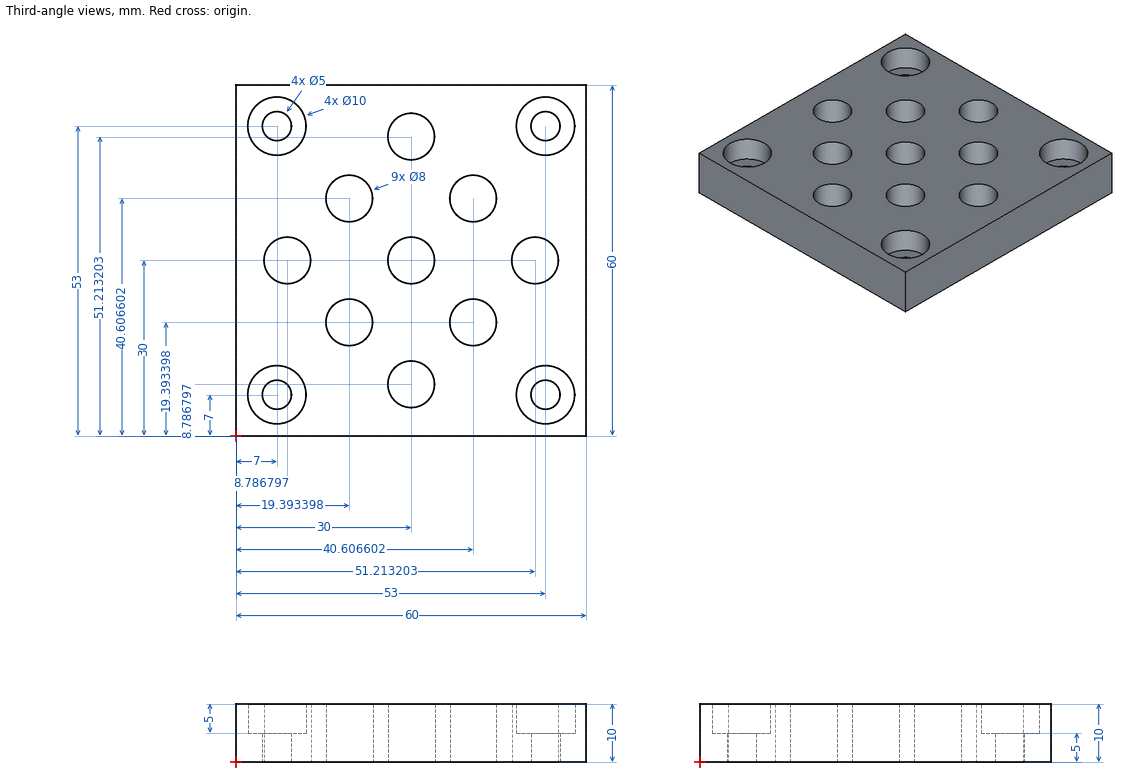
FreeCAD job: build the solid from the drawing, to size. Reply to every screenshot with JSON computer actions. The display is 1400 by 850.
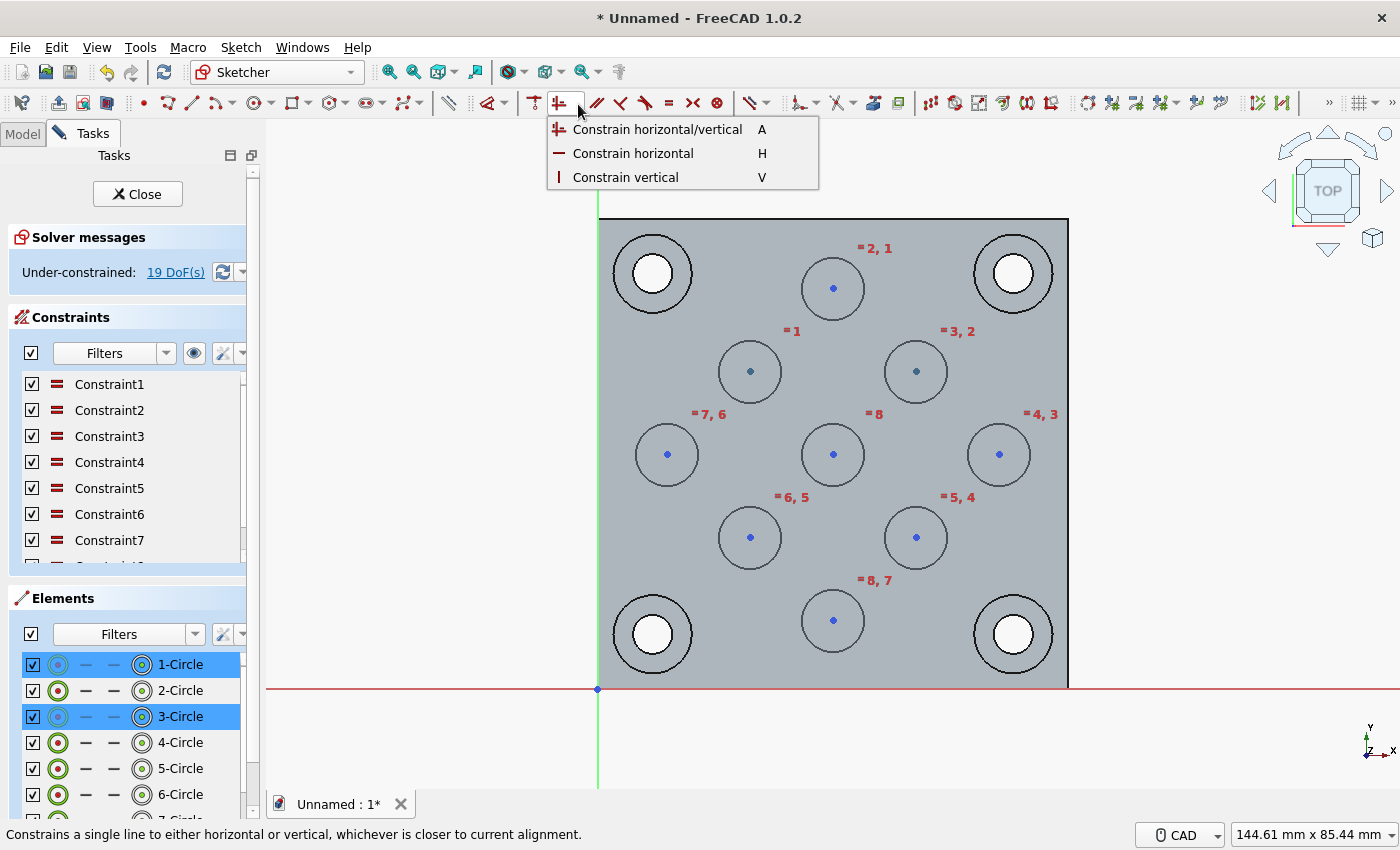
{"action": "left_click", "coordinate": [683, 153]}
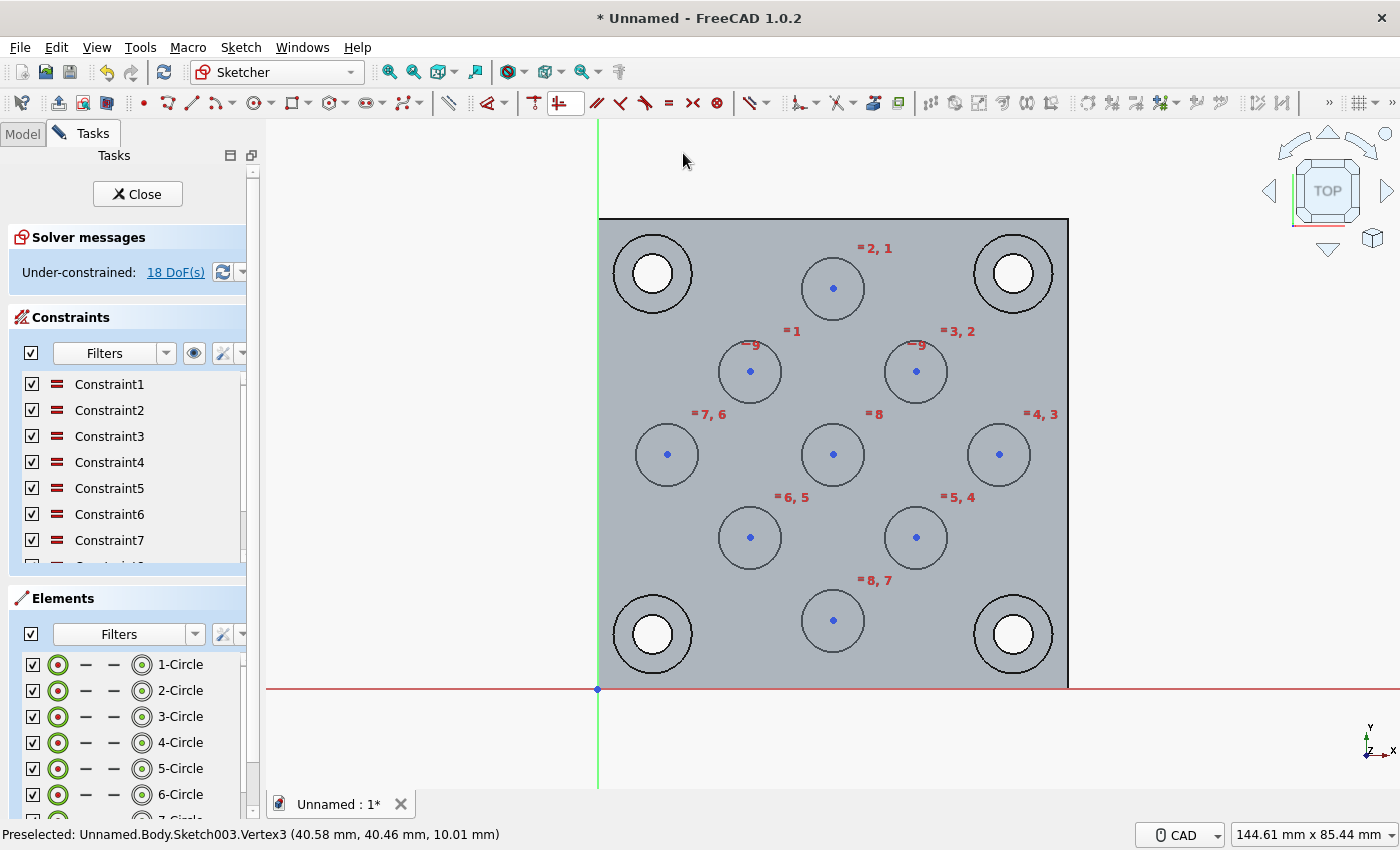
{"action": "left_click", "coordinate": [916, 372]}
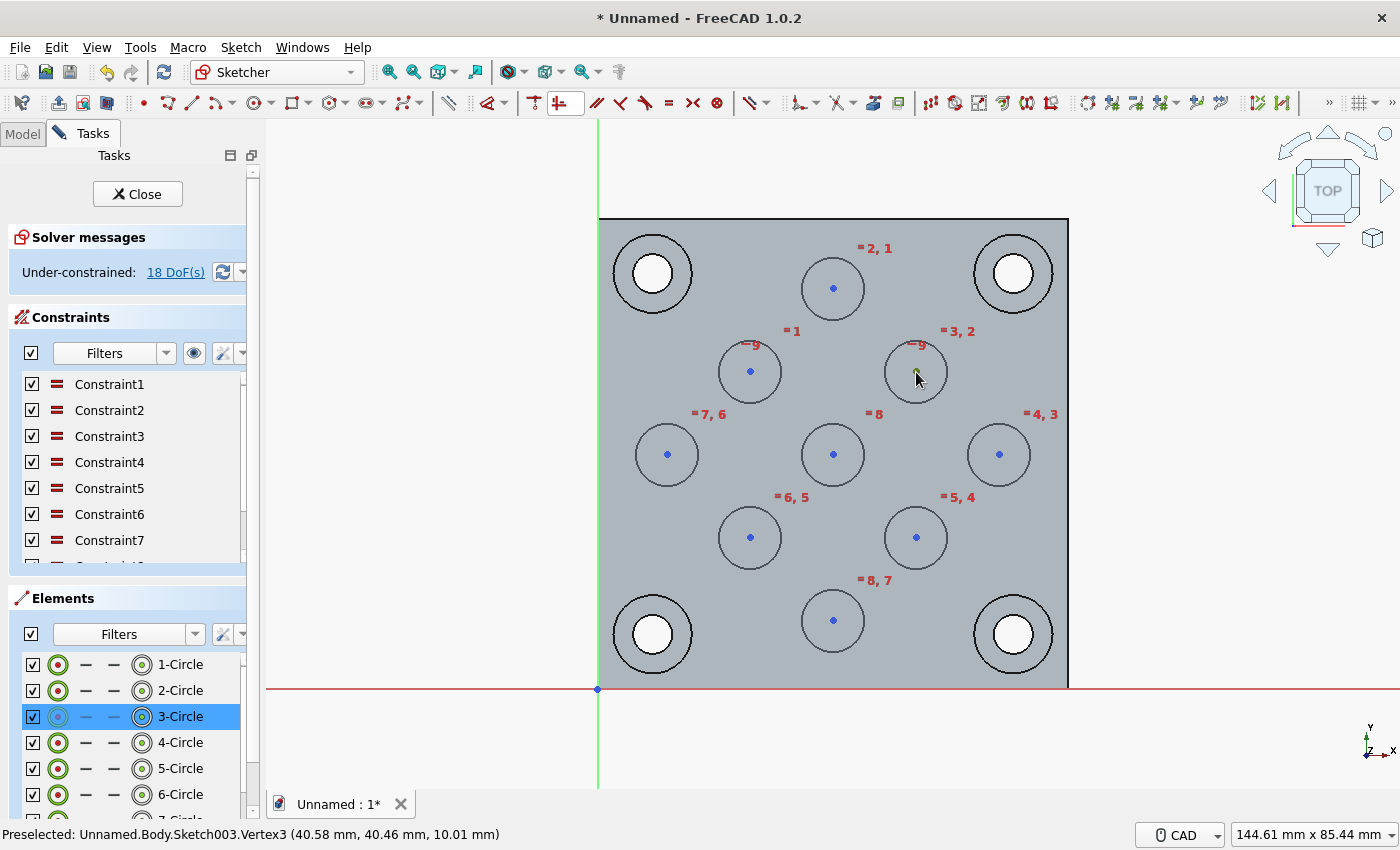
{"action": "left_click", "coordinate": [916, 538]}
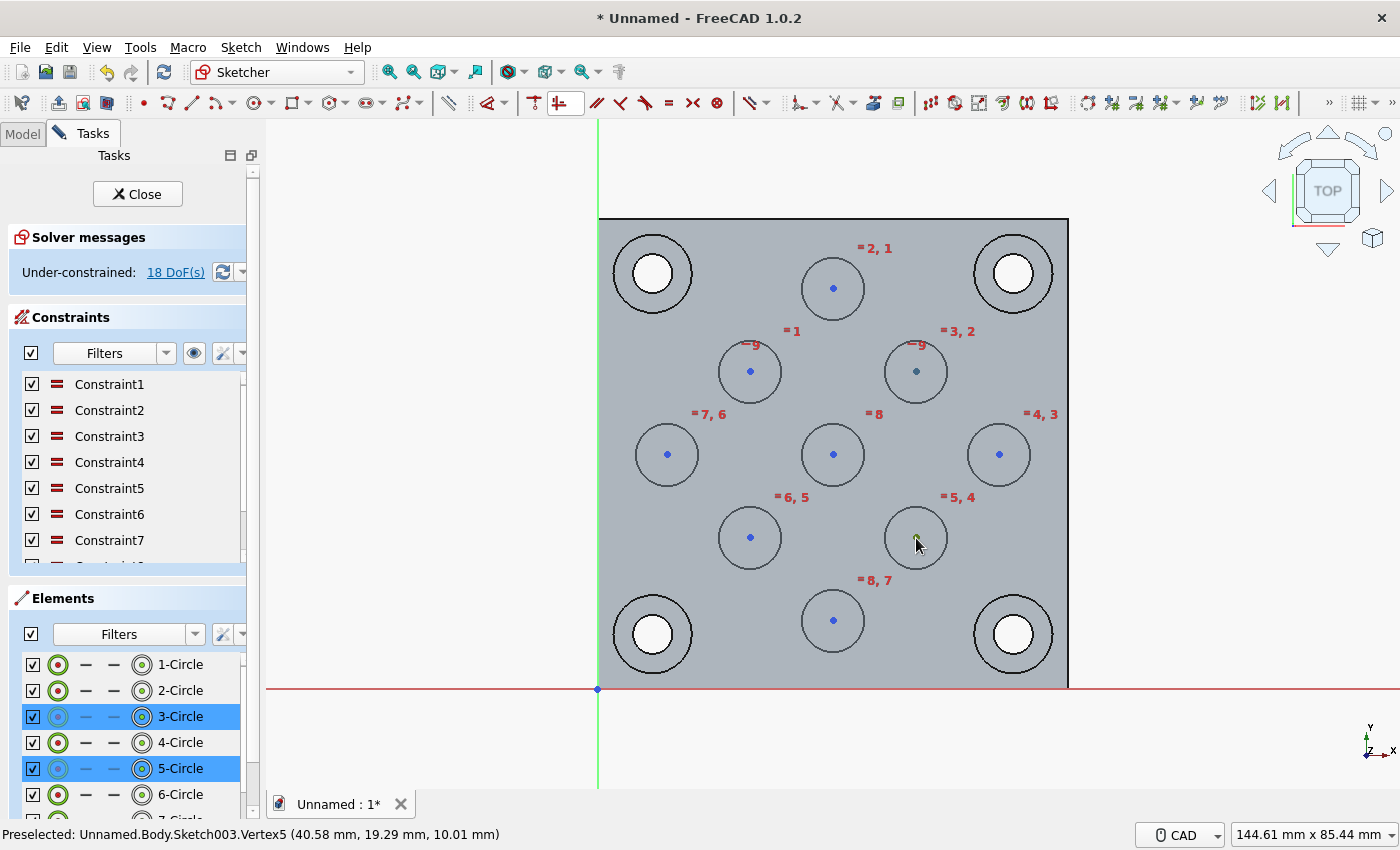
{"action": "left_click", "coordinate": [578, 104]}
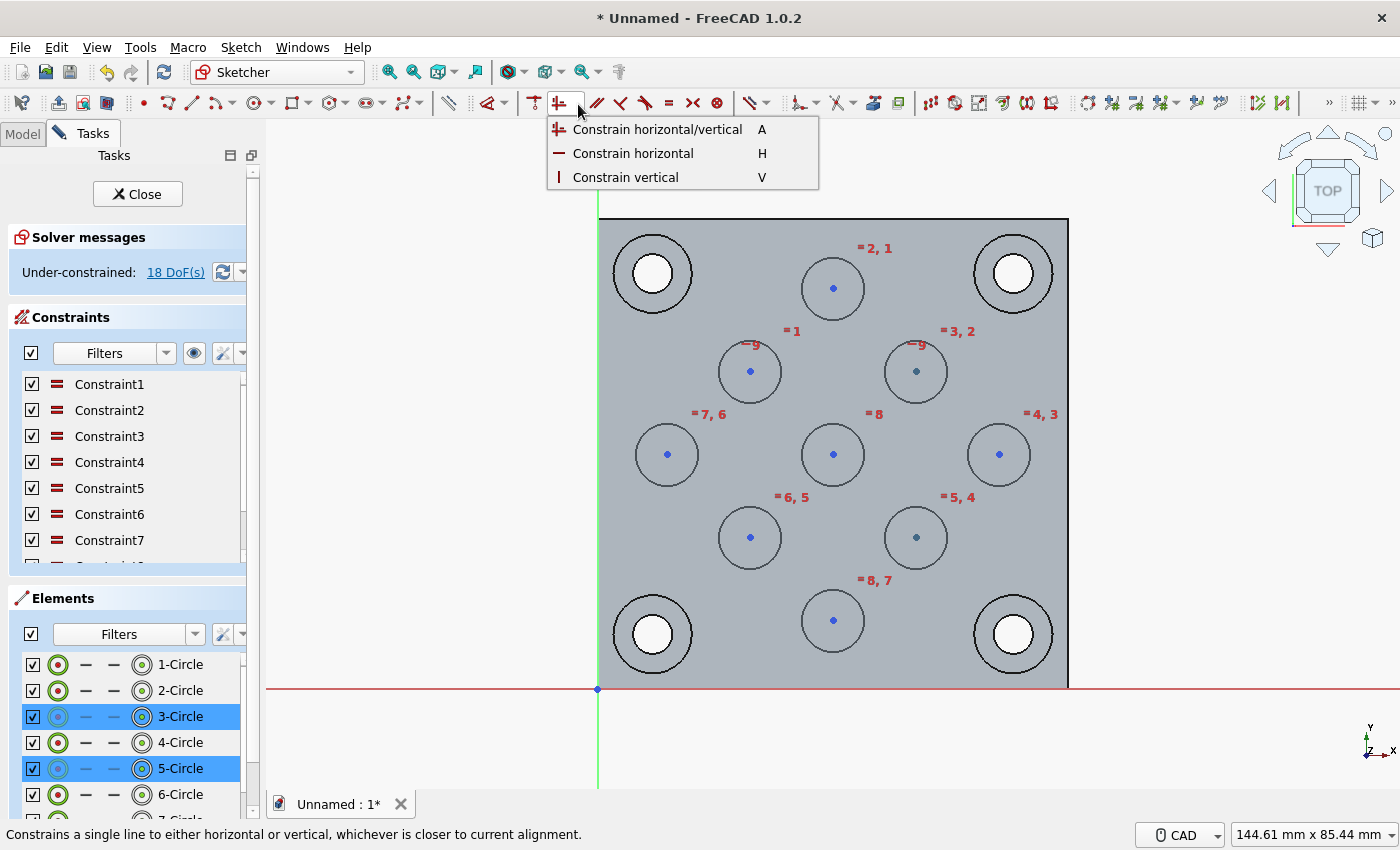
{"action": "left_click", "coordinate": [683, 177]}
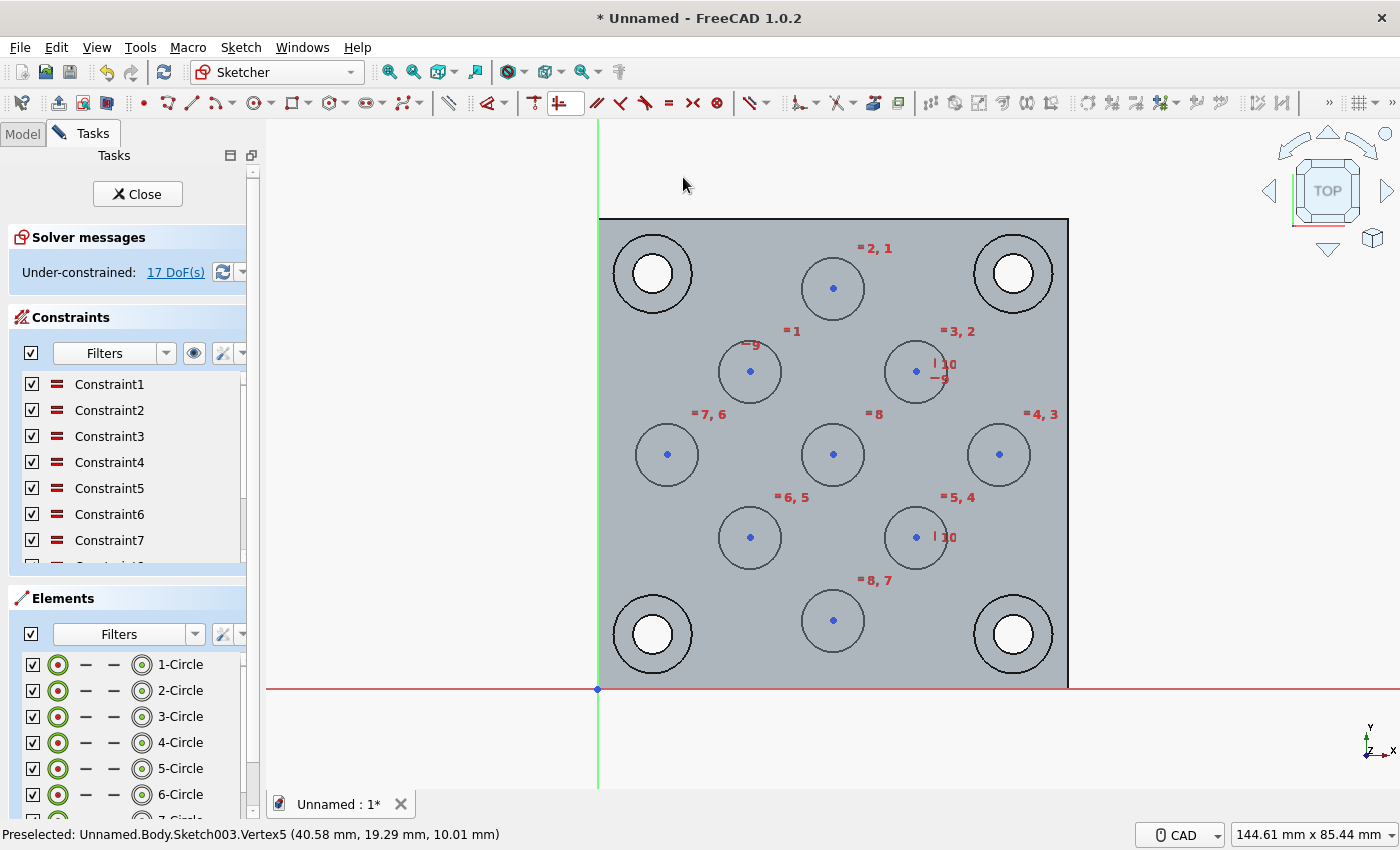
{"action": "left_click", "coordinate": [750, 372]}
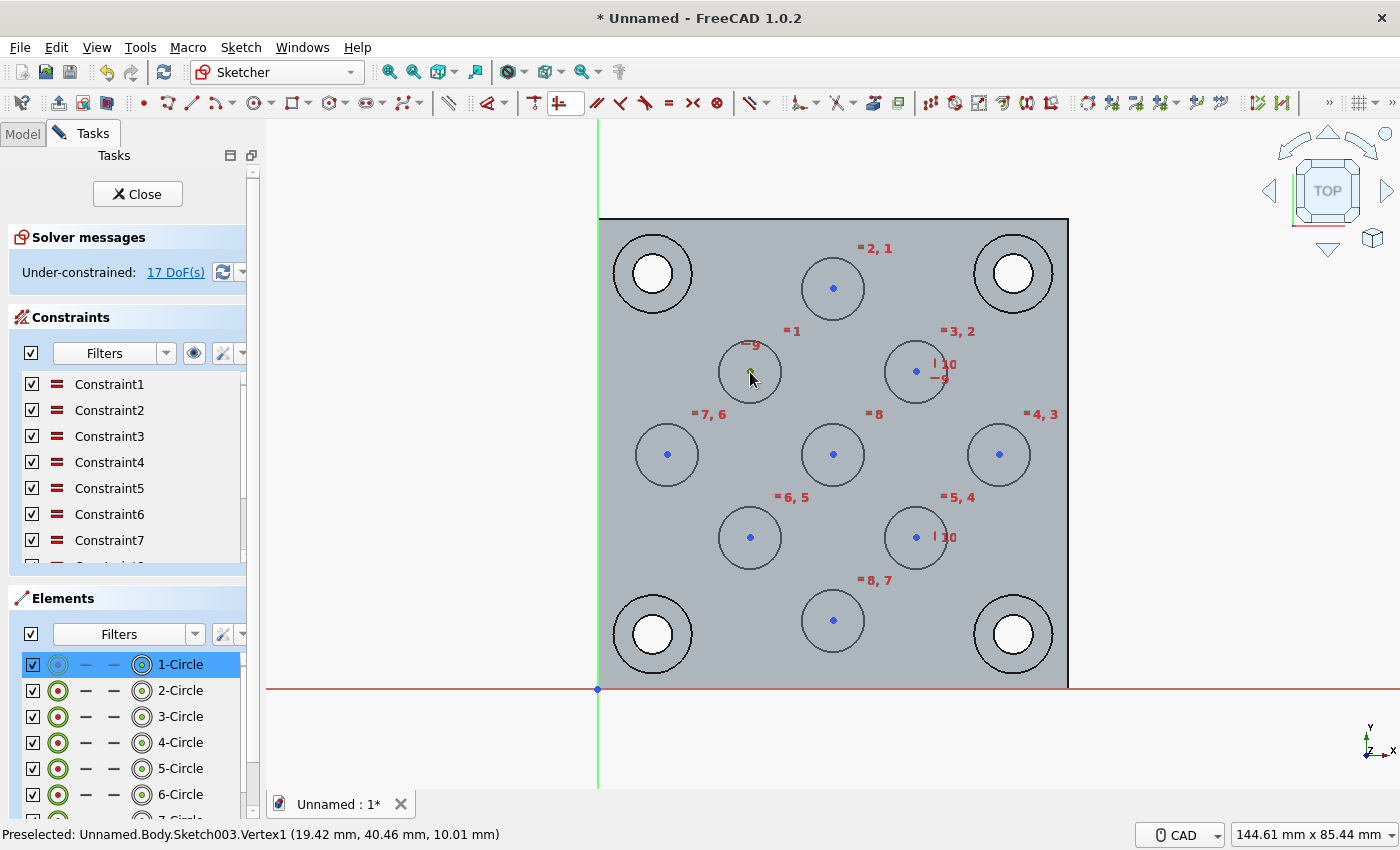
{"action": "left_click", "coordinate": [750, 538]}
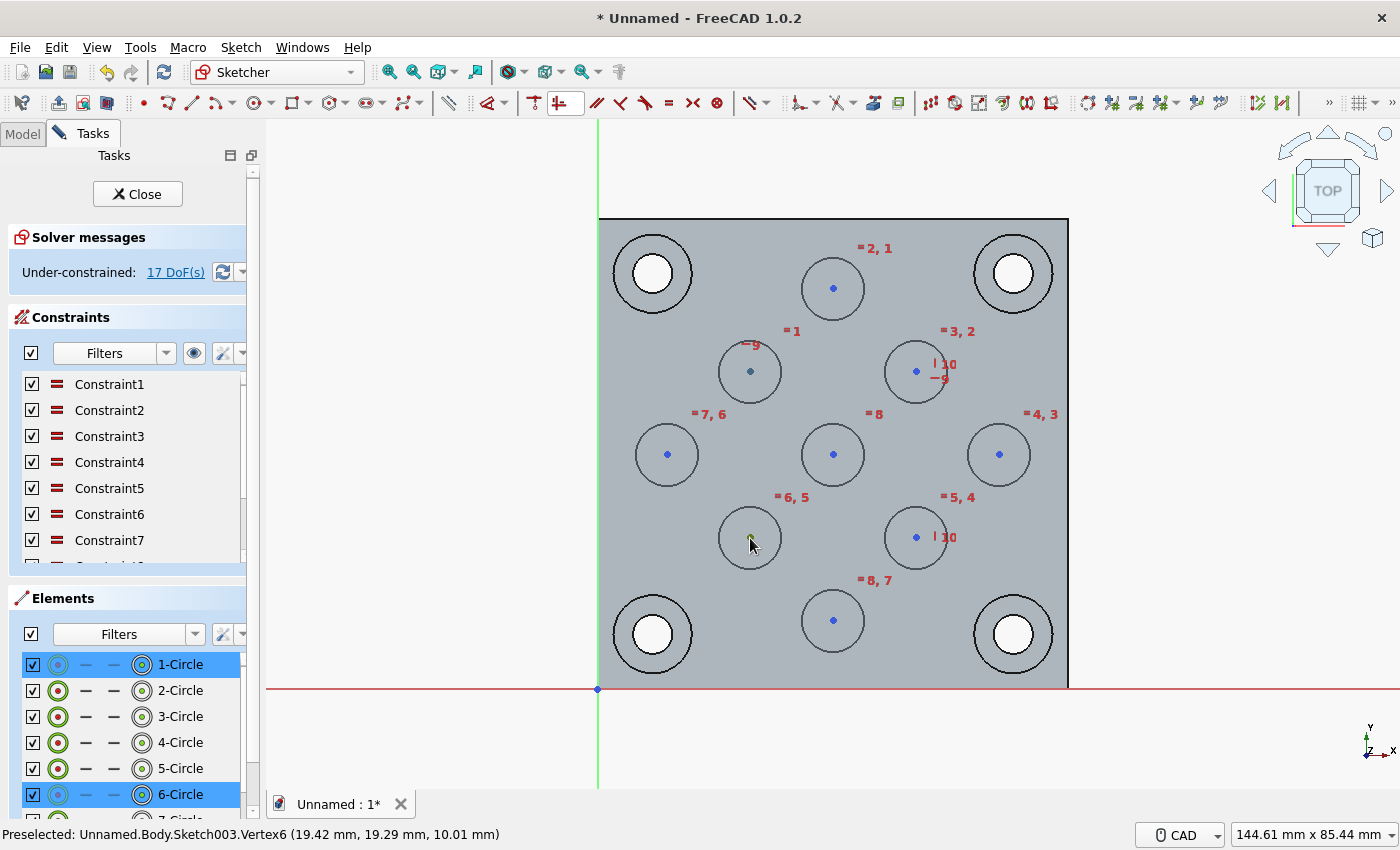
{"action": "key", "text": "v"}